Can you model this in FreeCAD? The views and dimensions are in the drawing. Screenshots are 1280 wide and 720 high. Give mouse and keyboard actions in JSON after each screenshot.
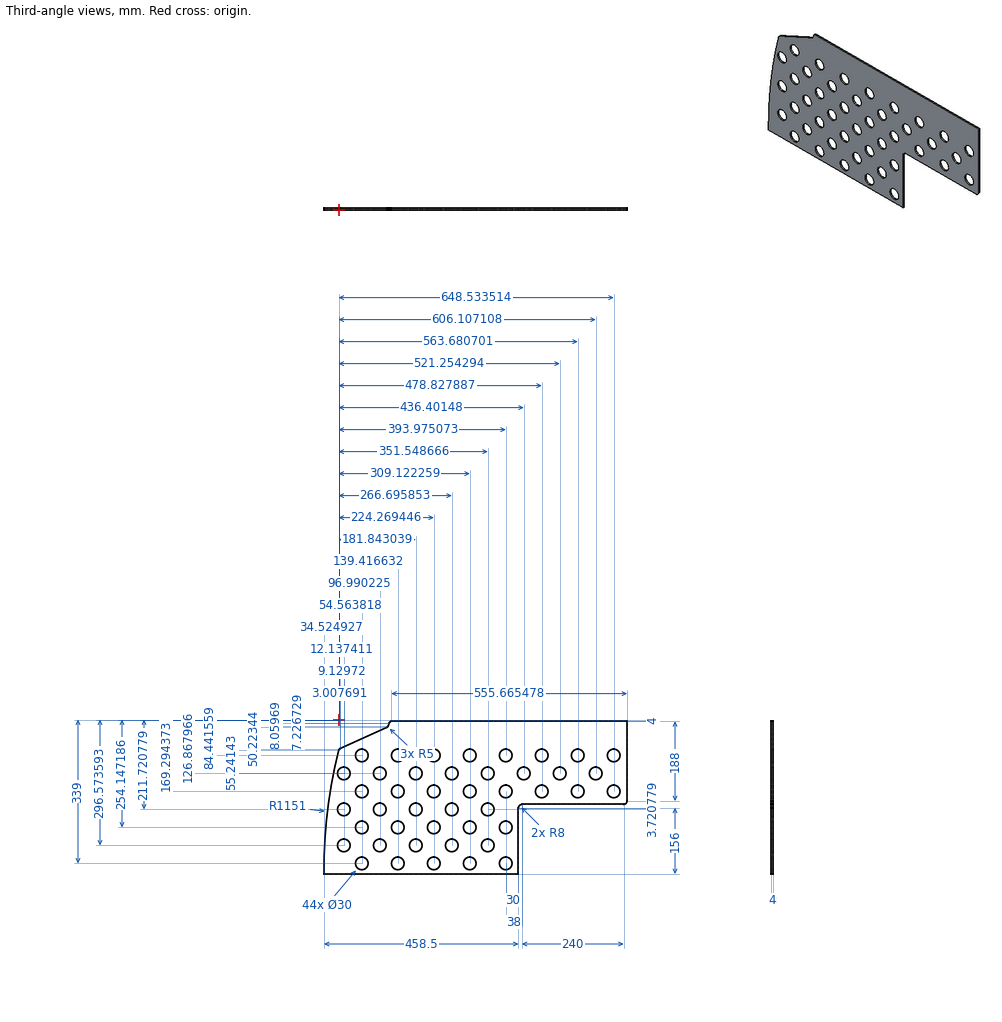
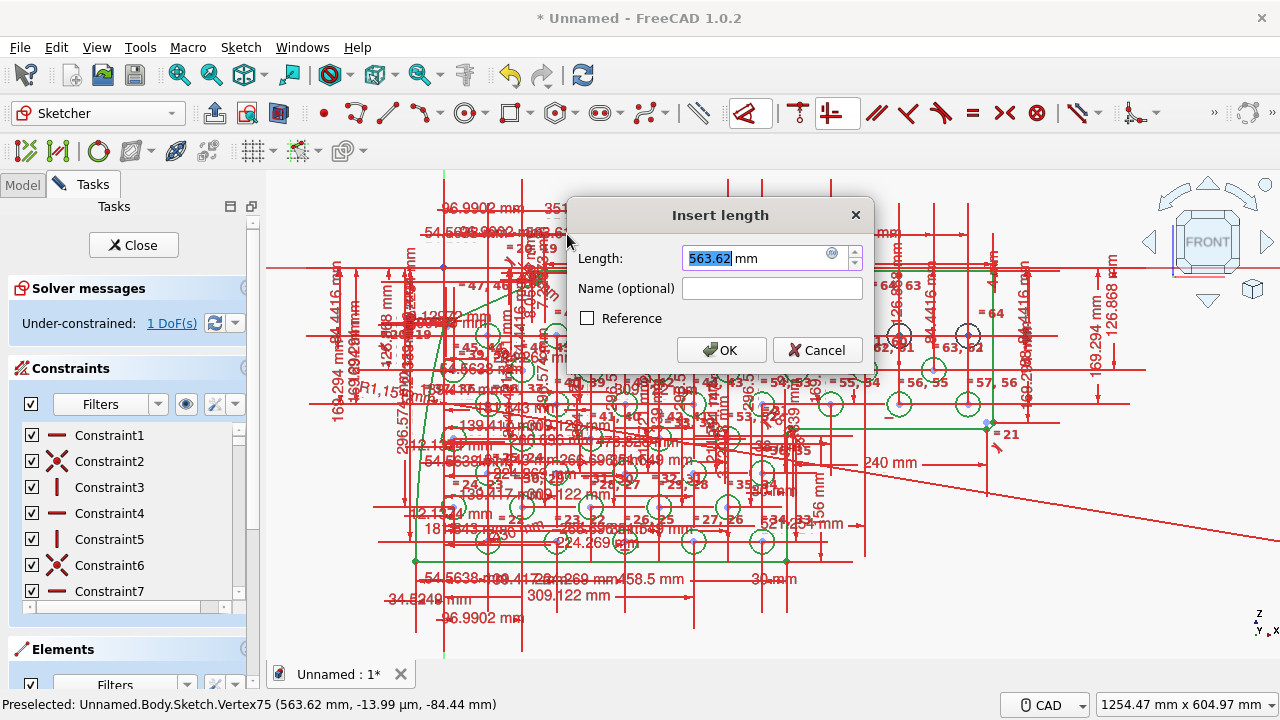
{"action": "type", "text": "563.680701"}
{"action": "key", "text": "Return"}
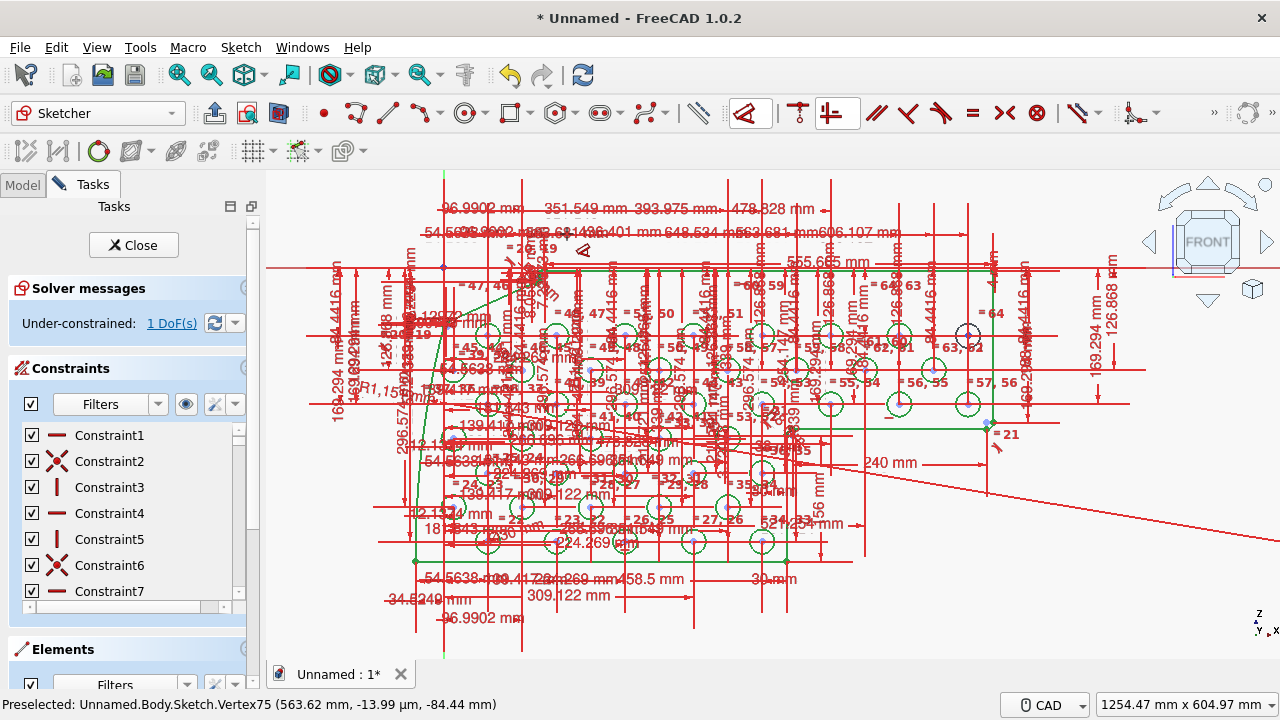
{"action": "left_click", "coordinate": [968, 336]}
{"action": "left_click", "coordinate": [890, 210]}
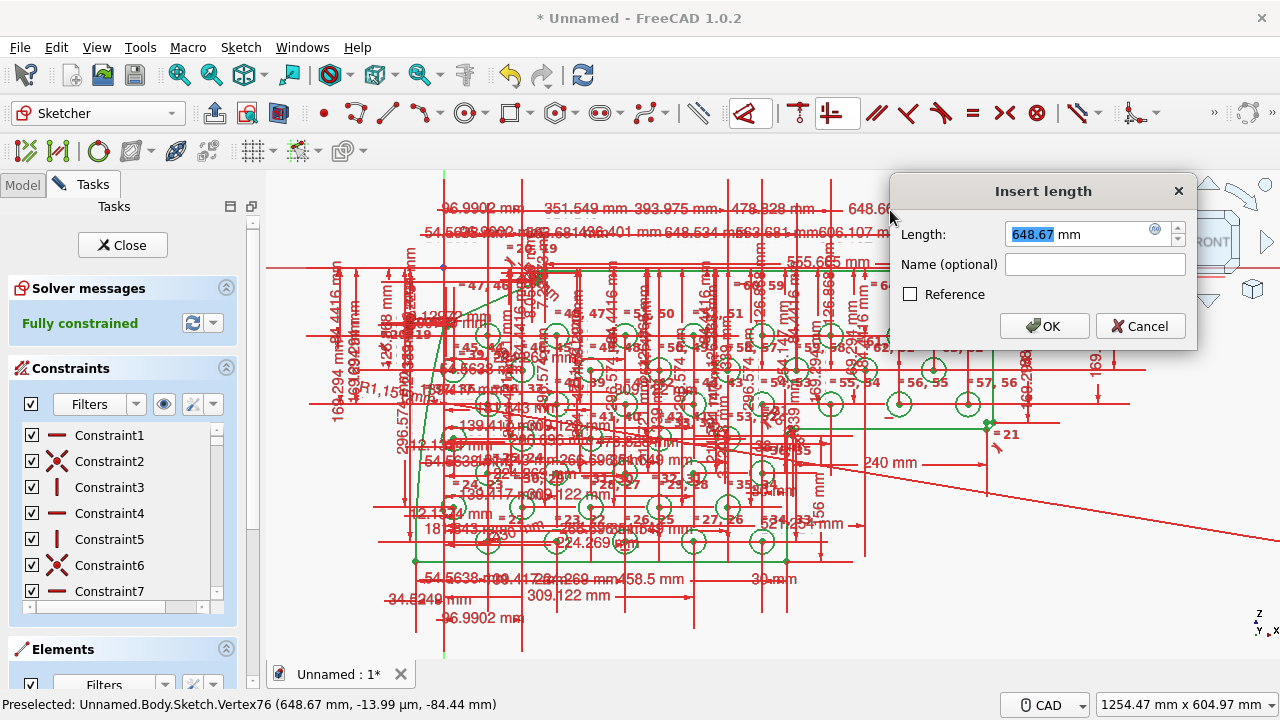
{"action": "type", "text": "648.533514"}
{"action": "key", "text": "Return"}
{"action": "key", "text": "Escape"}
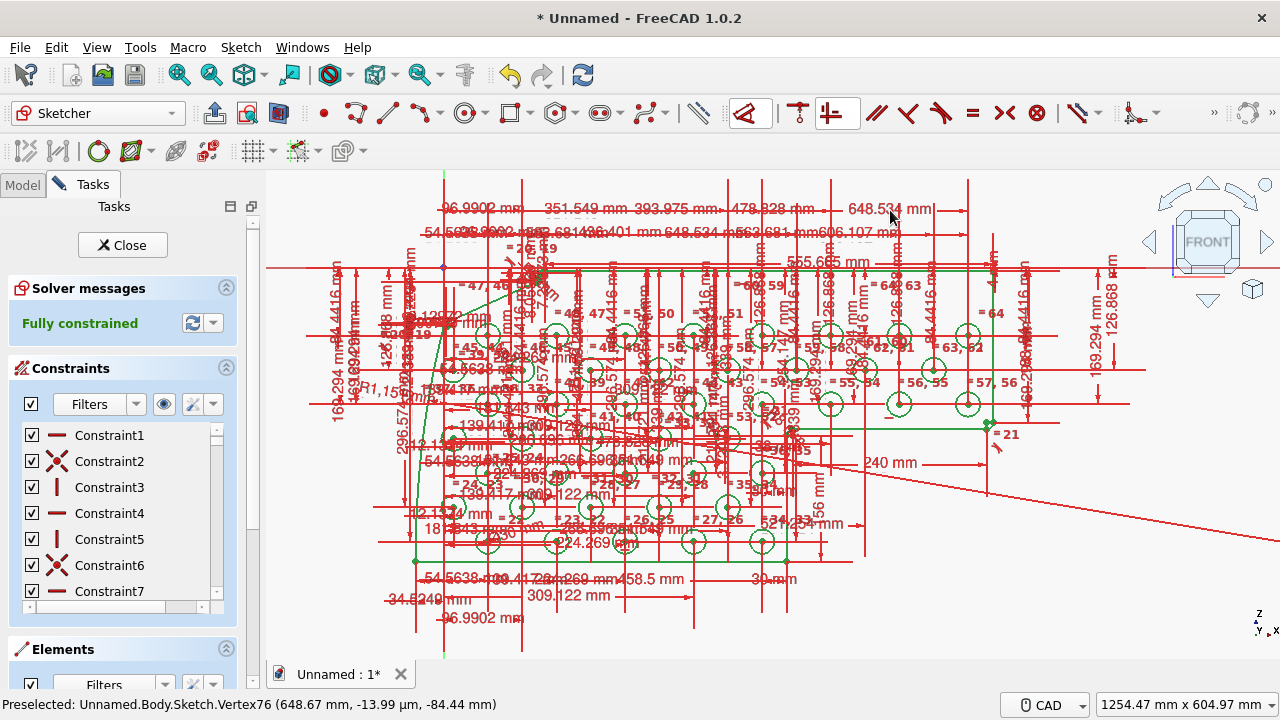
{"action": "left_click", "coordinate": [123, 245]}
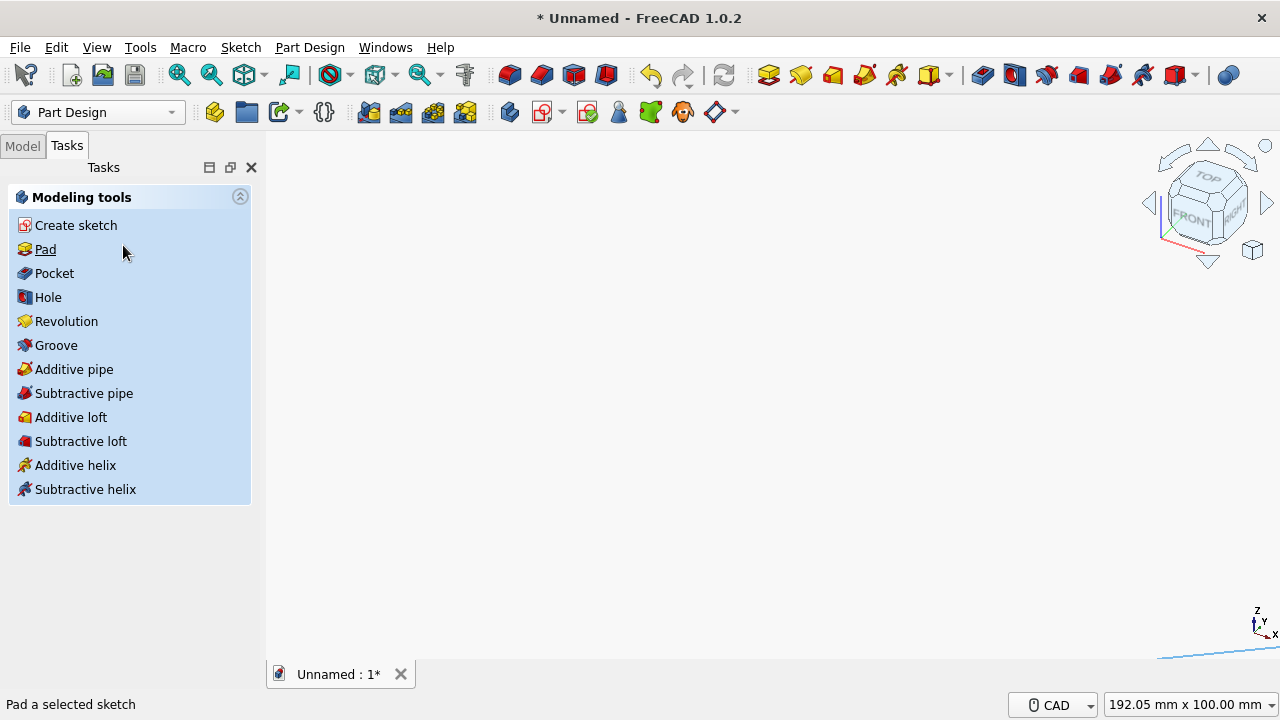
{"action": "left_click", "coordinate": [770, 76]}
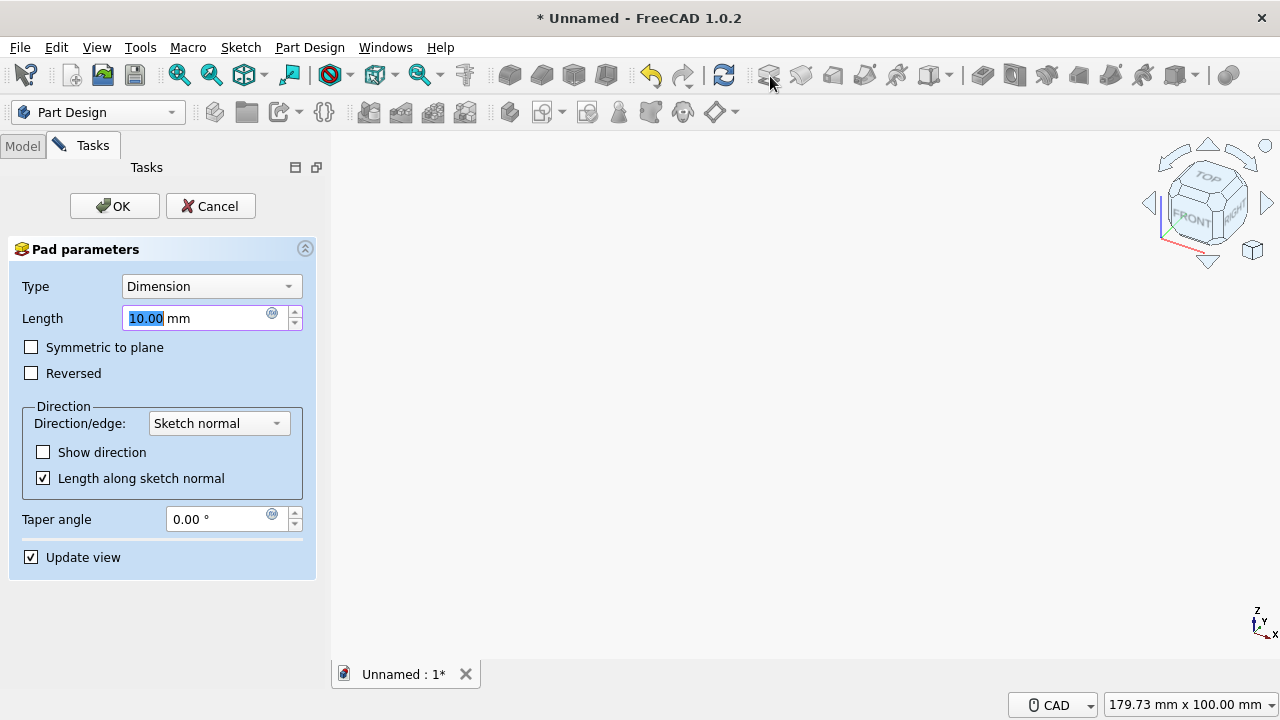
{"action": "type", "text": "4"}
{"action": "key", "text": "Tab"}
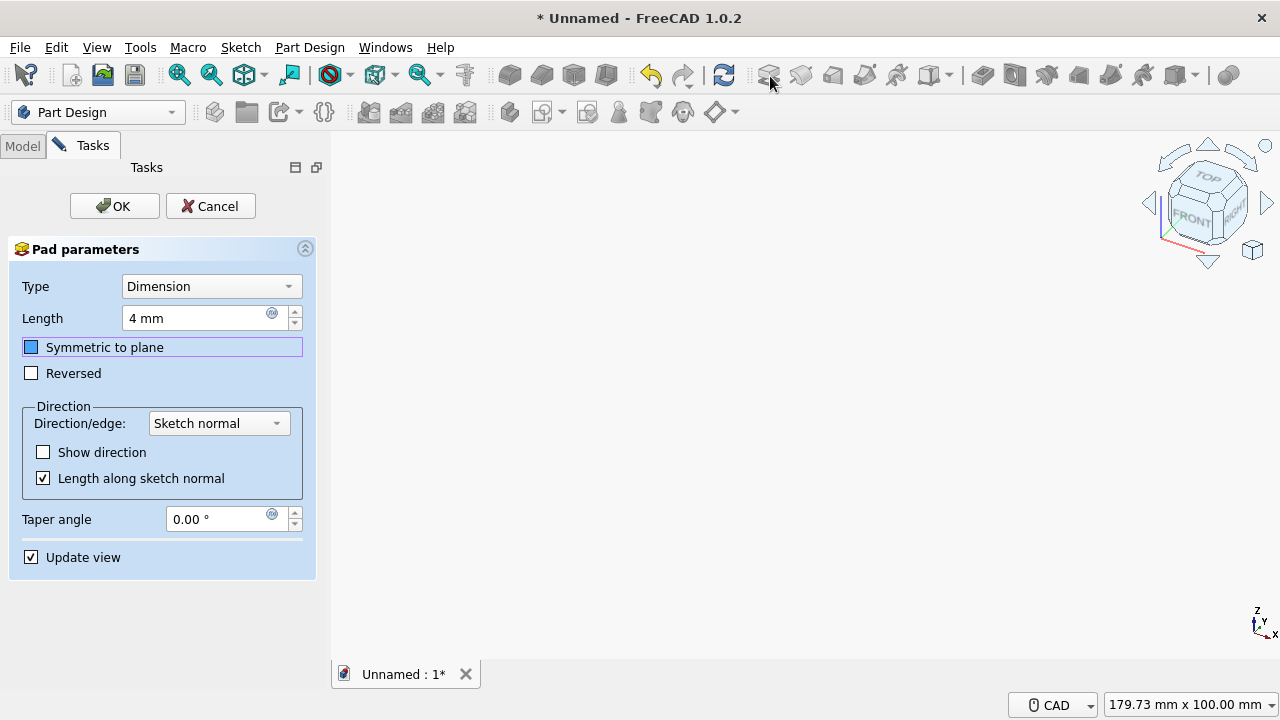
{"action": "left_click", "coordinate": [30, 373]}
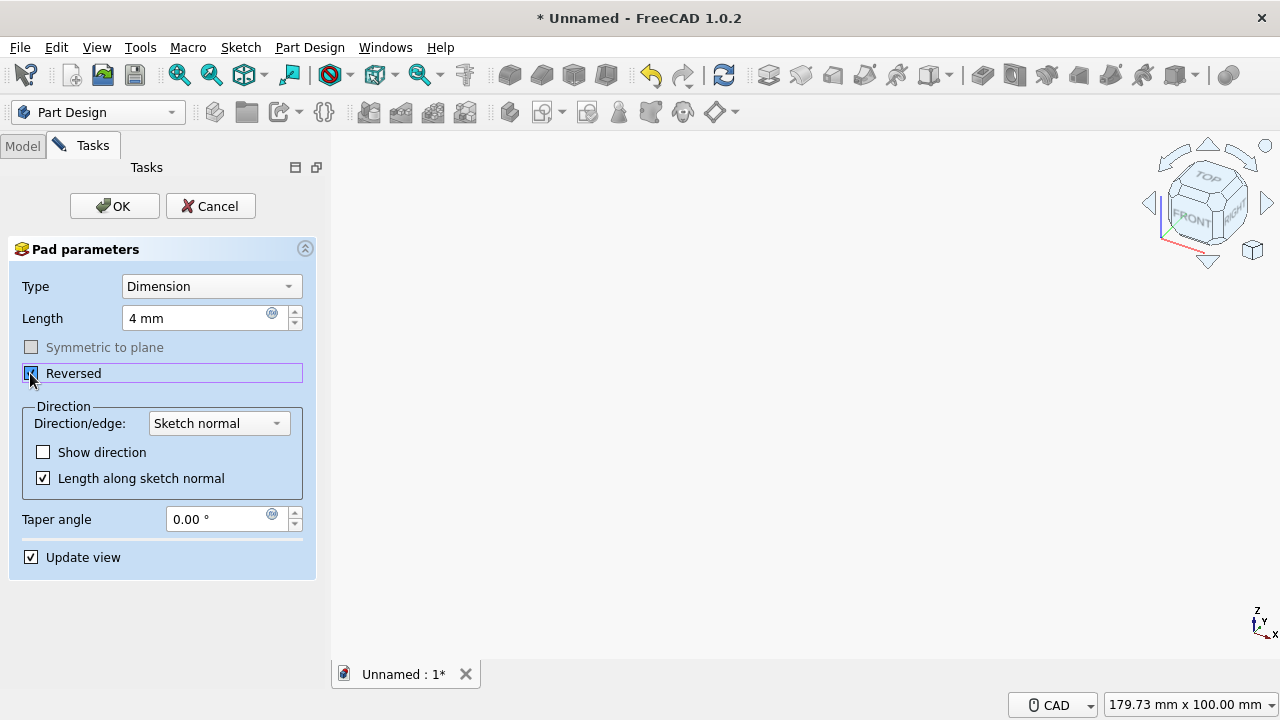
{"action": "left_click", "coordinate": [115, 206]}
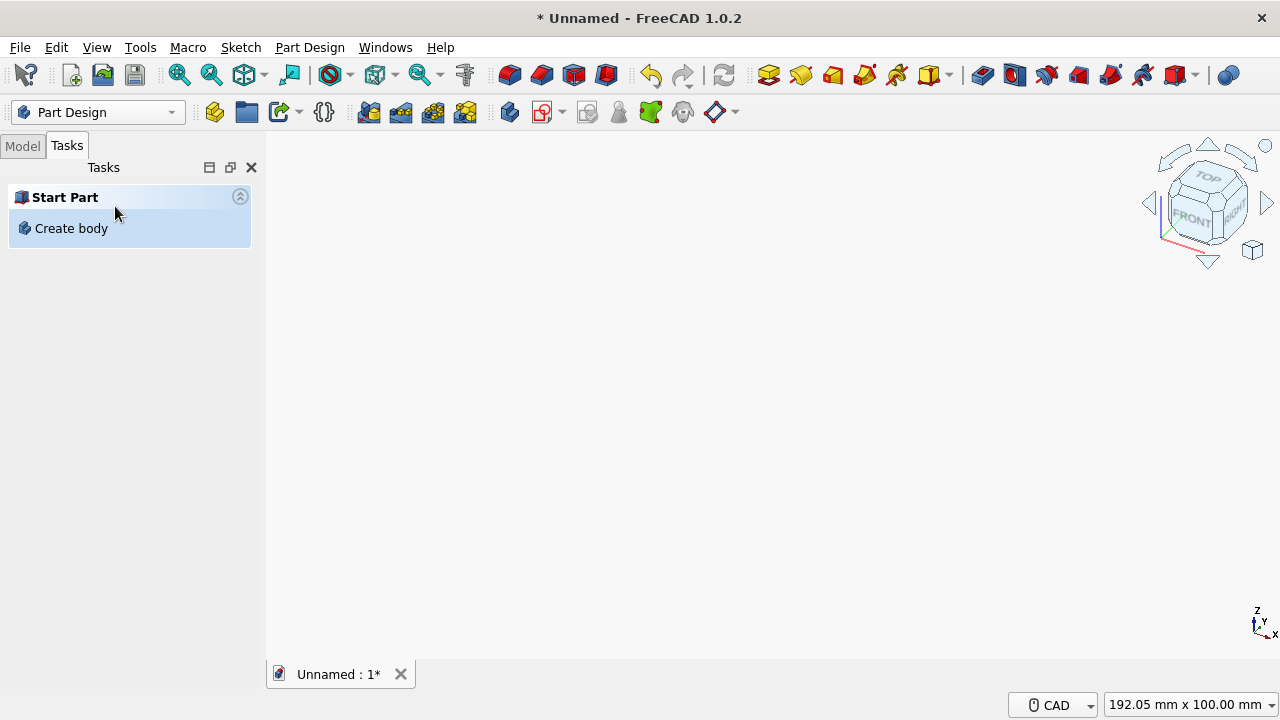
{"action": "key", "text": "0"}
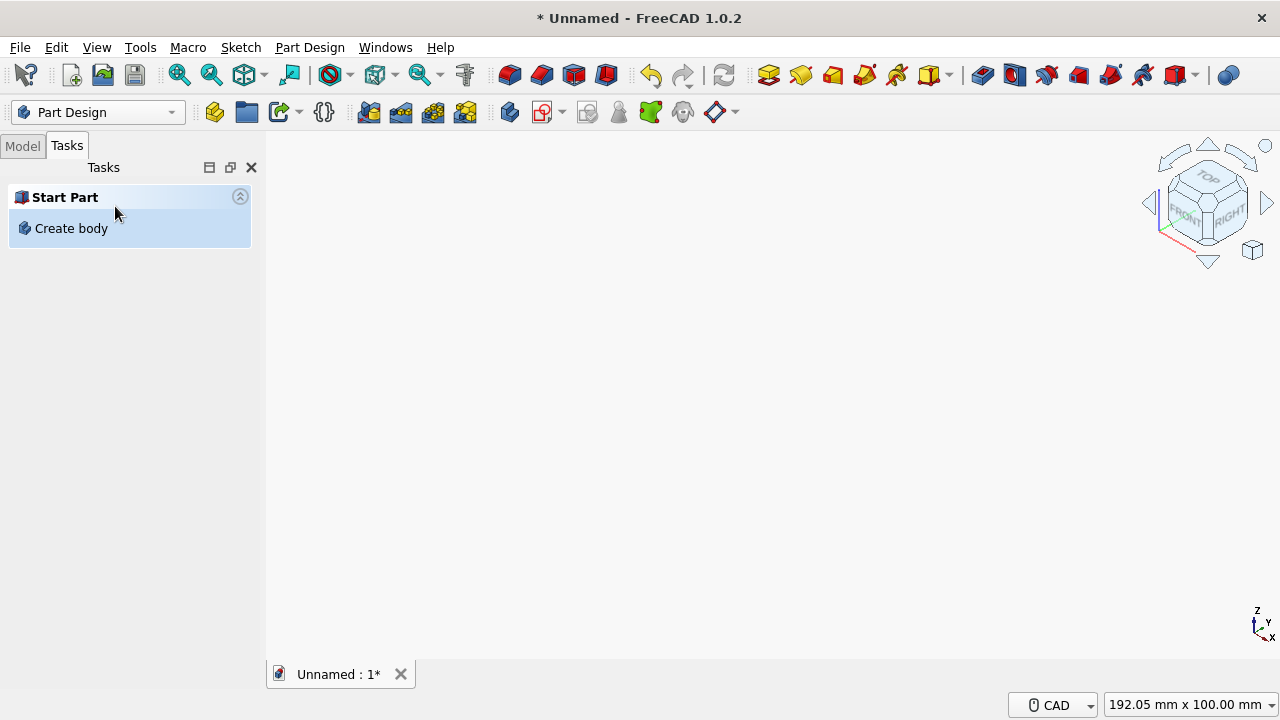
{"action": "key", "text": "v f"}